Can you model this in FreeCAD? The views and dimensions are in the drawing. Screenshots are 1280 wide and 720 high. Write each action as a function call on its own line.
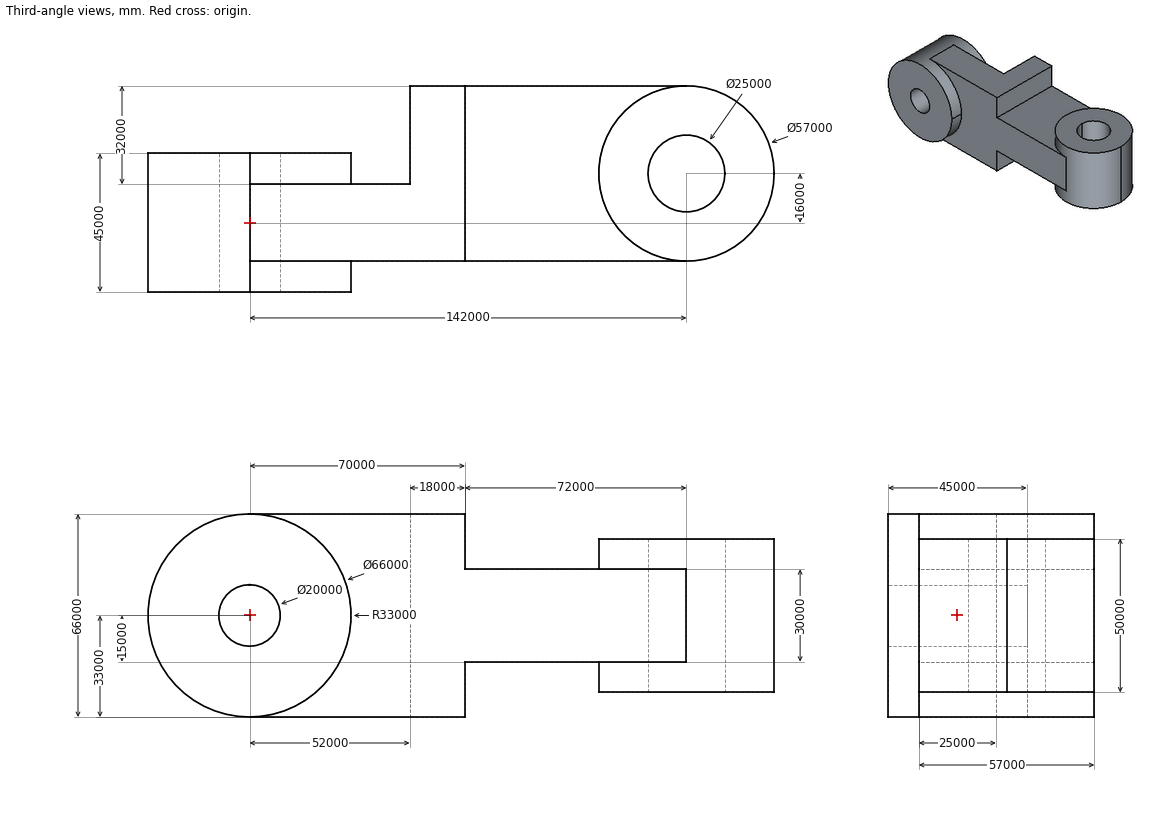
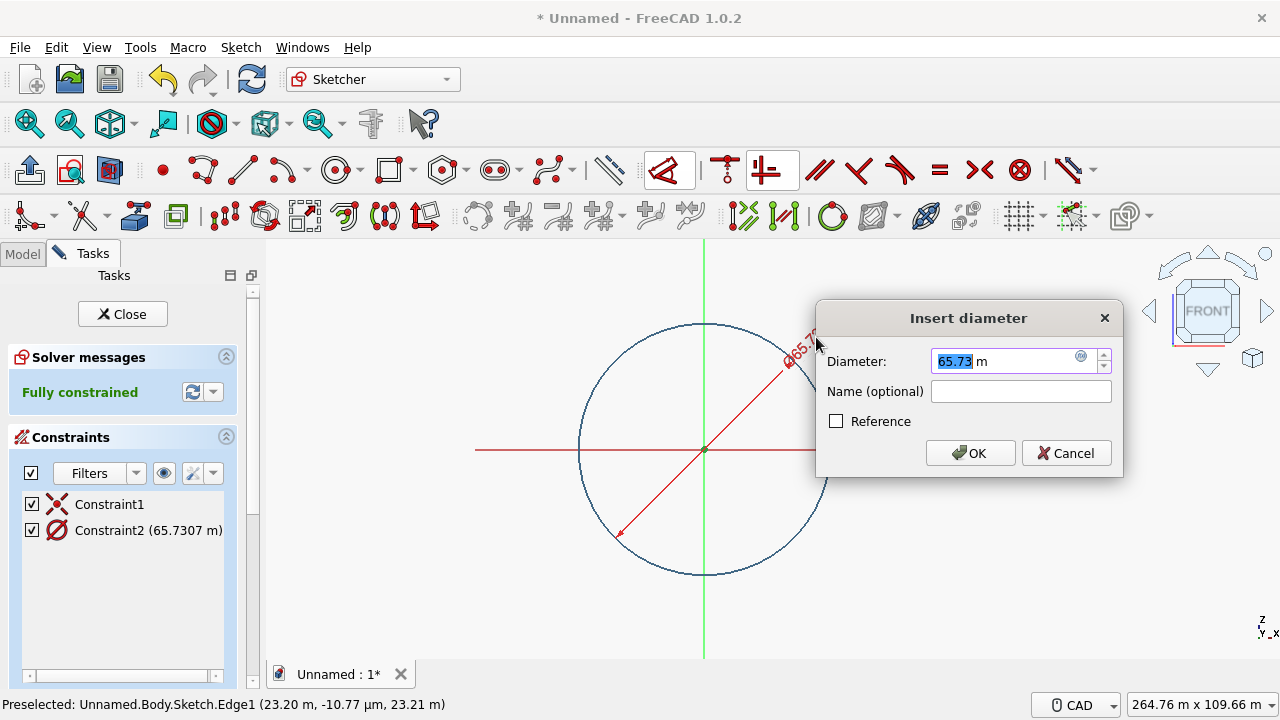
key(ctrl+a)
text(66000 mm)
key(Return)
key(Escape)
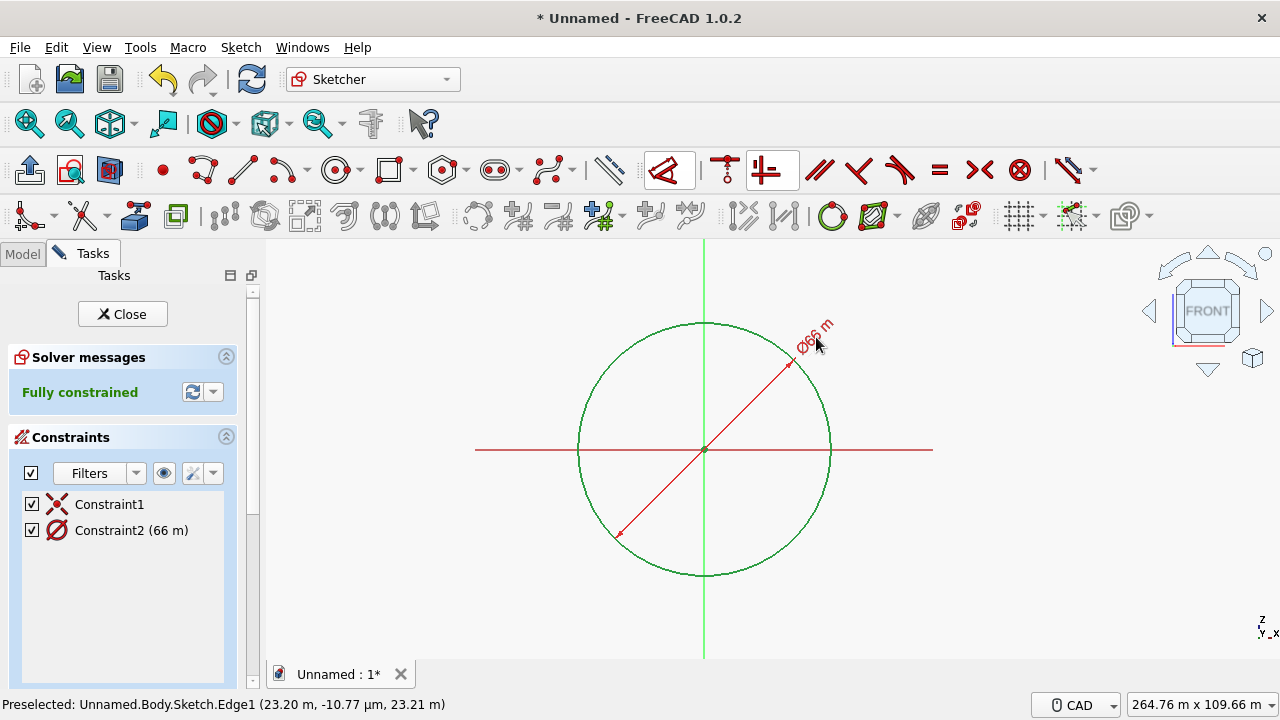
click(123, 314)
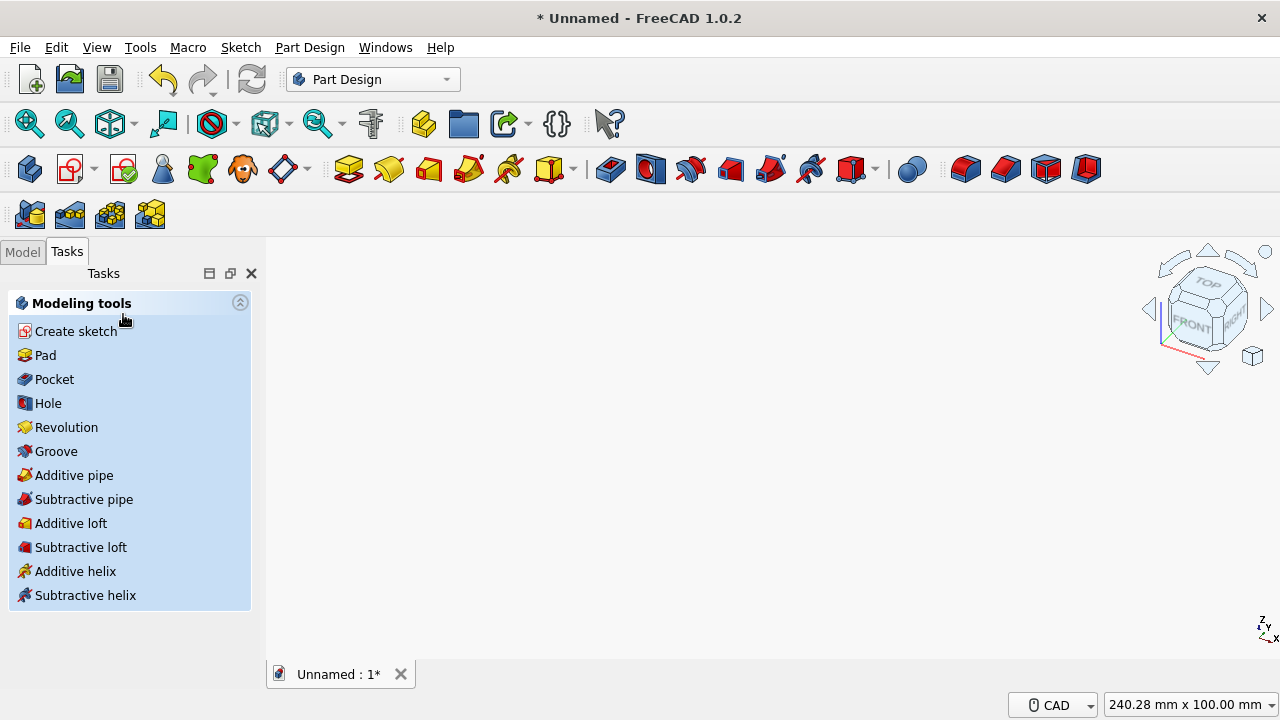
click(350, 170)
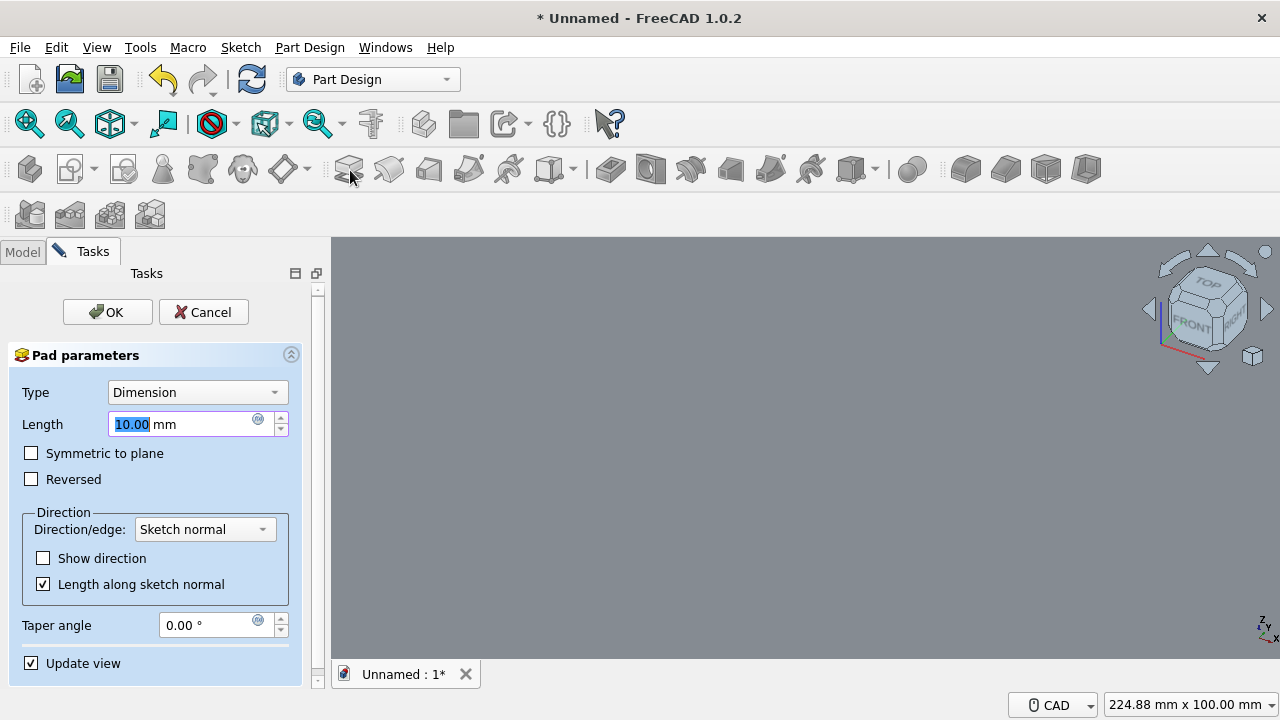
text(45000)
key(Tab)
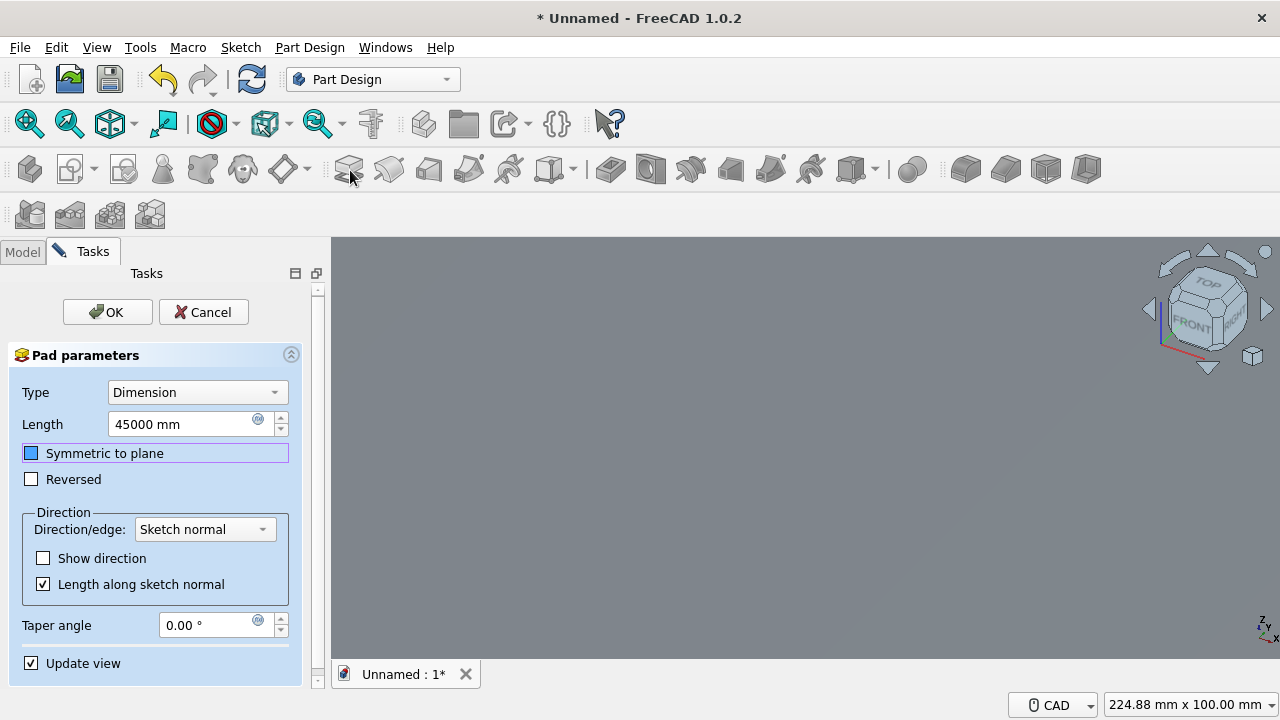
click(30, 453)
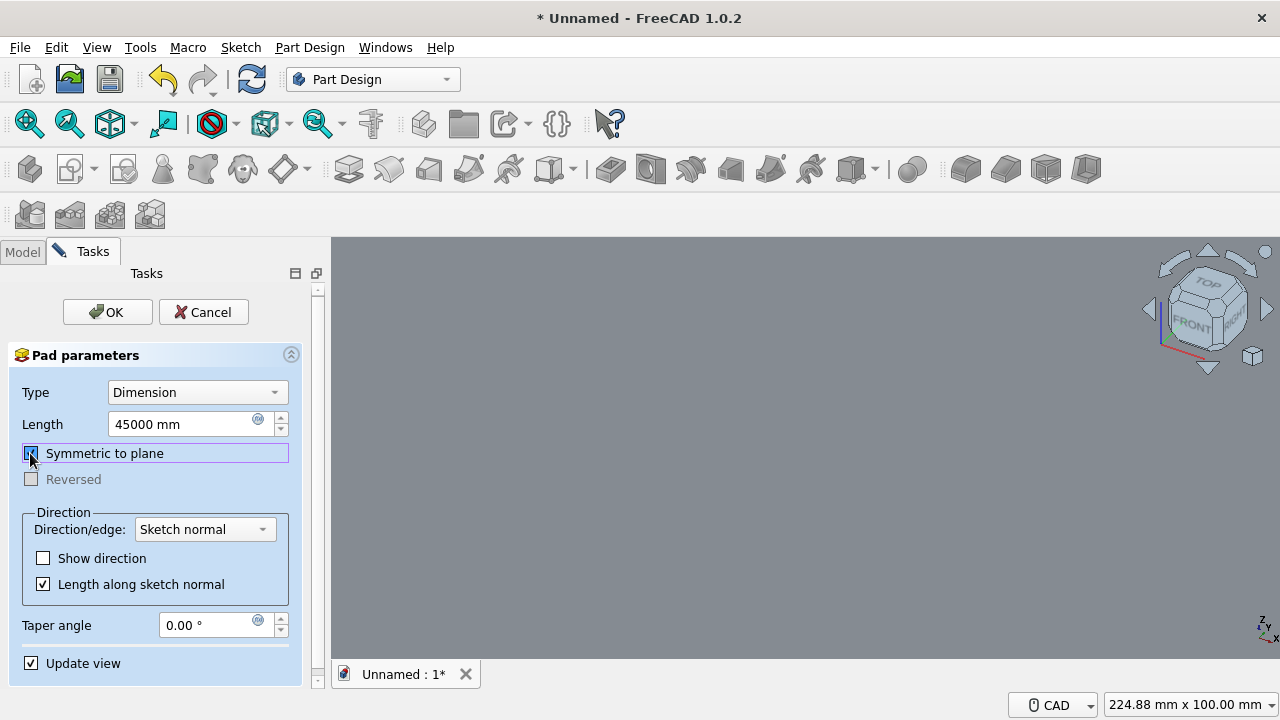
click(108, 312)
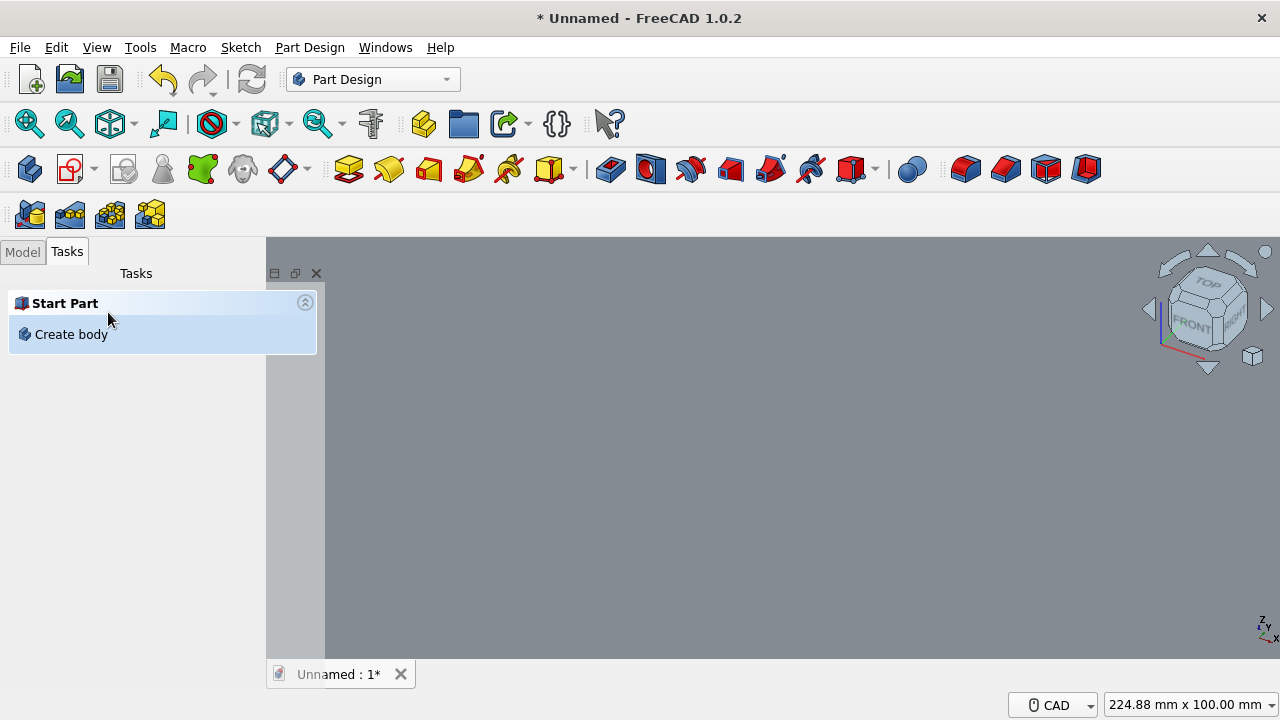
click(30, 124)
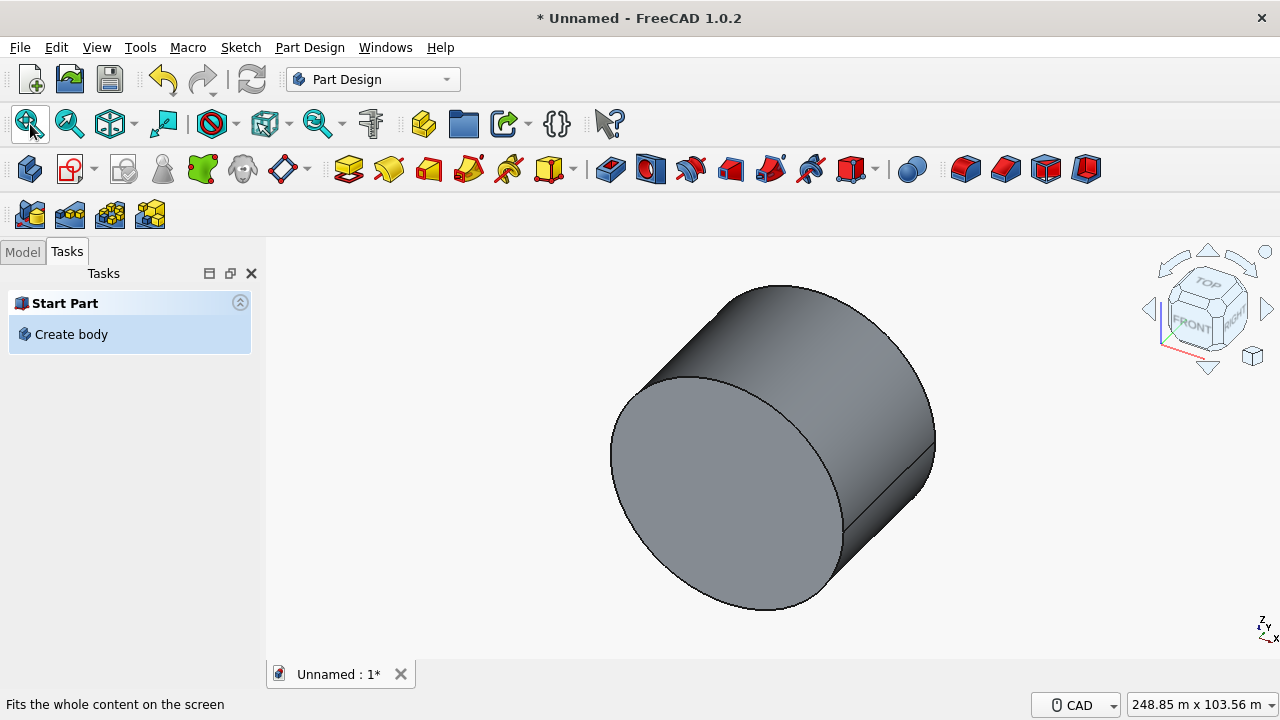
key(4)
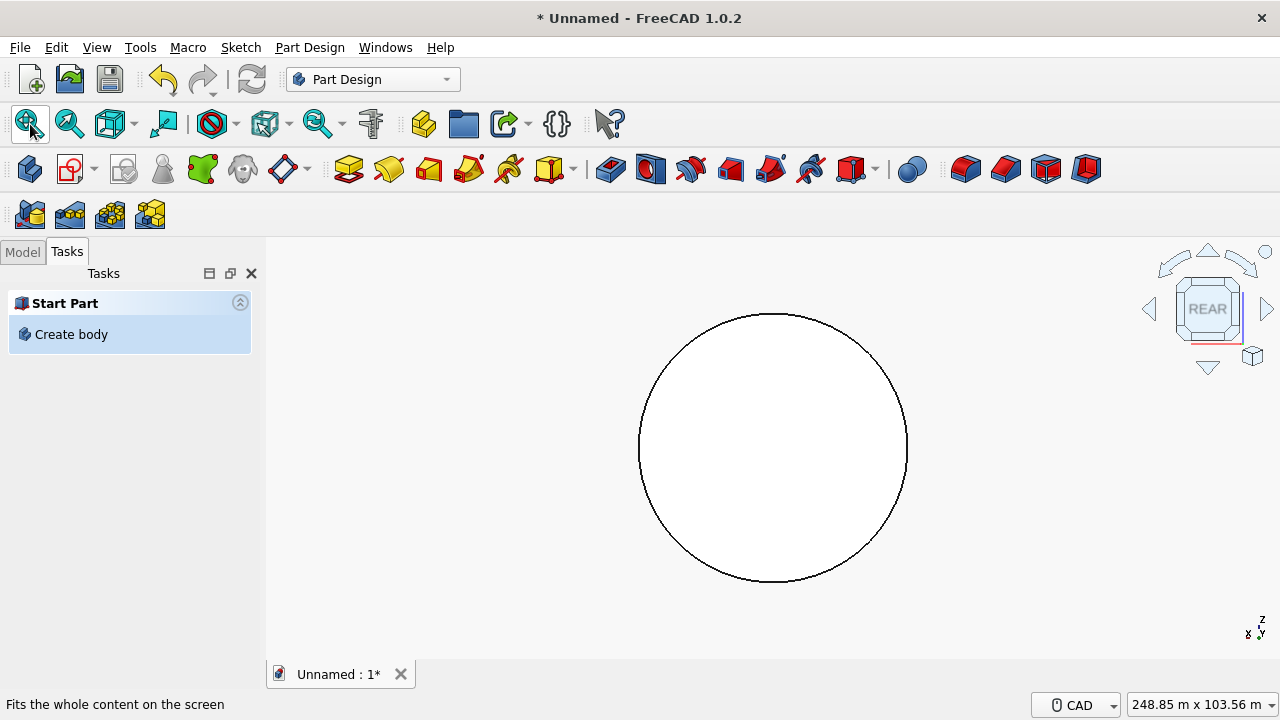
click(773, 447)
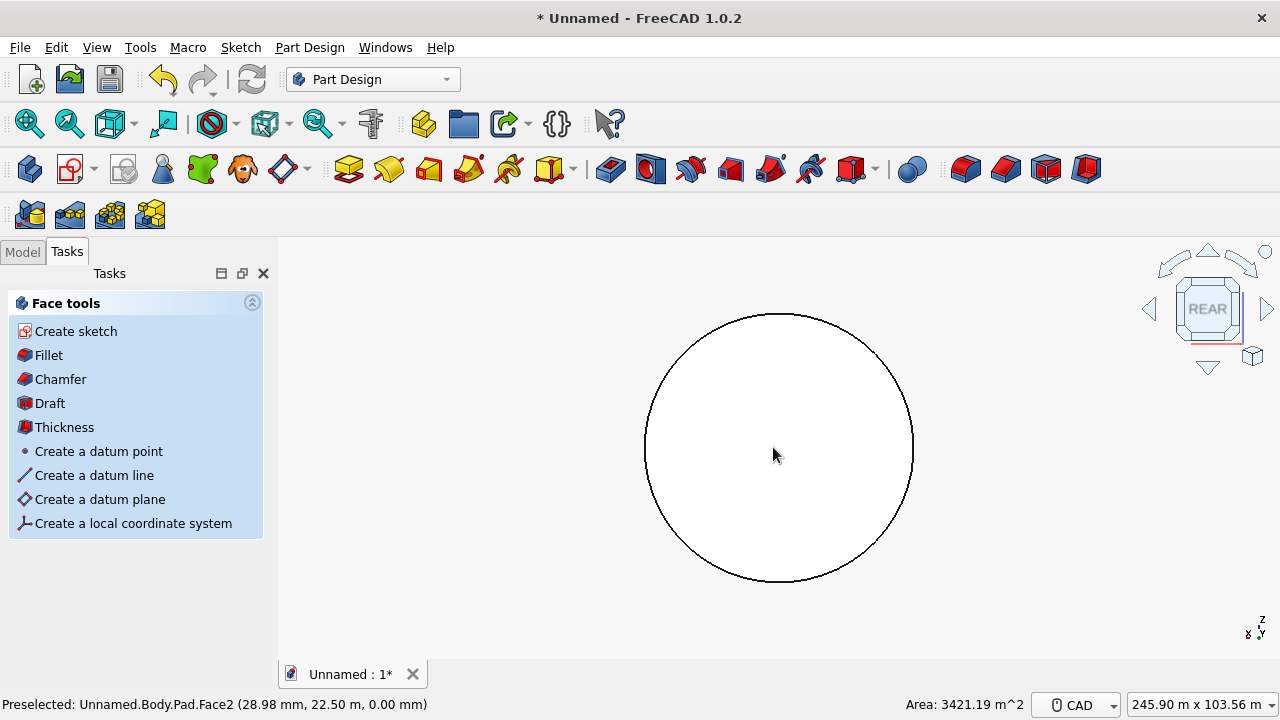
click(70, 170)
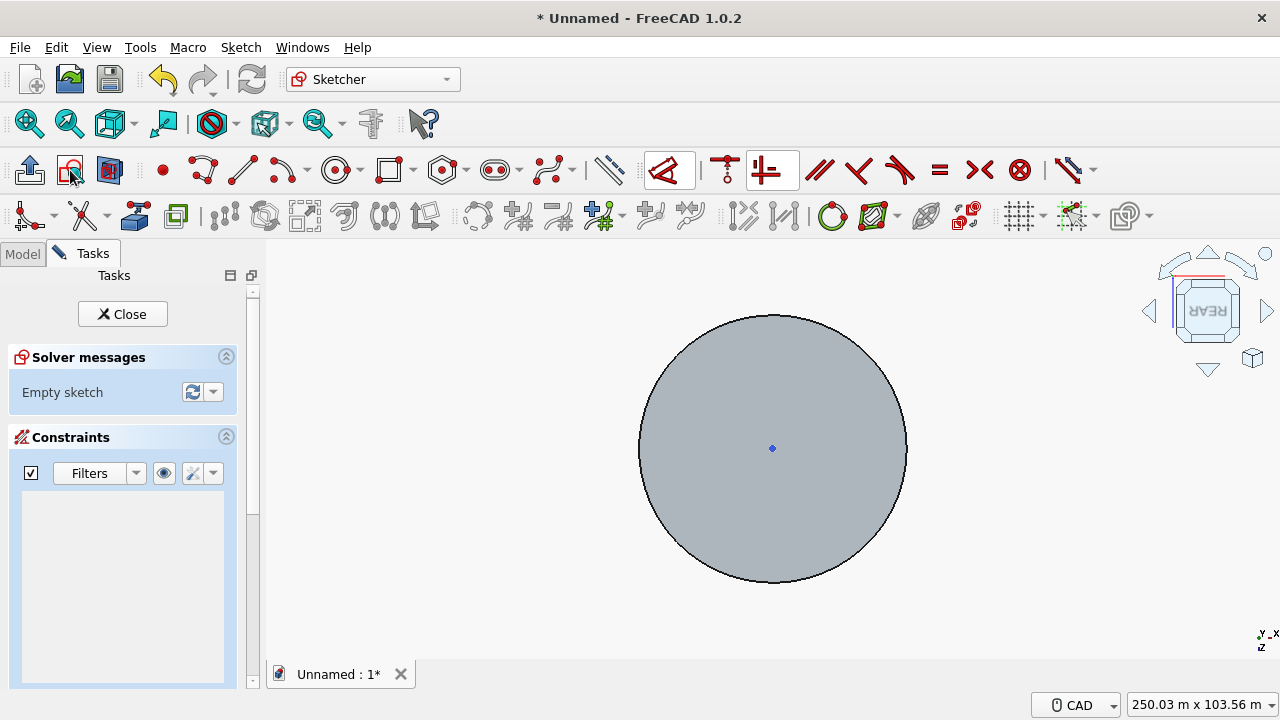
scroll(802, 449, up, 6)